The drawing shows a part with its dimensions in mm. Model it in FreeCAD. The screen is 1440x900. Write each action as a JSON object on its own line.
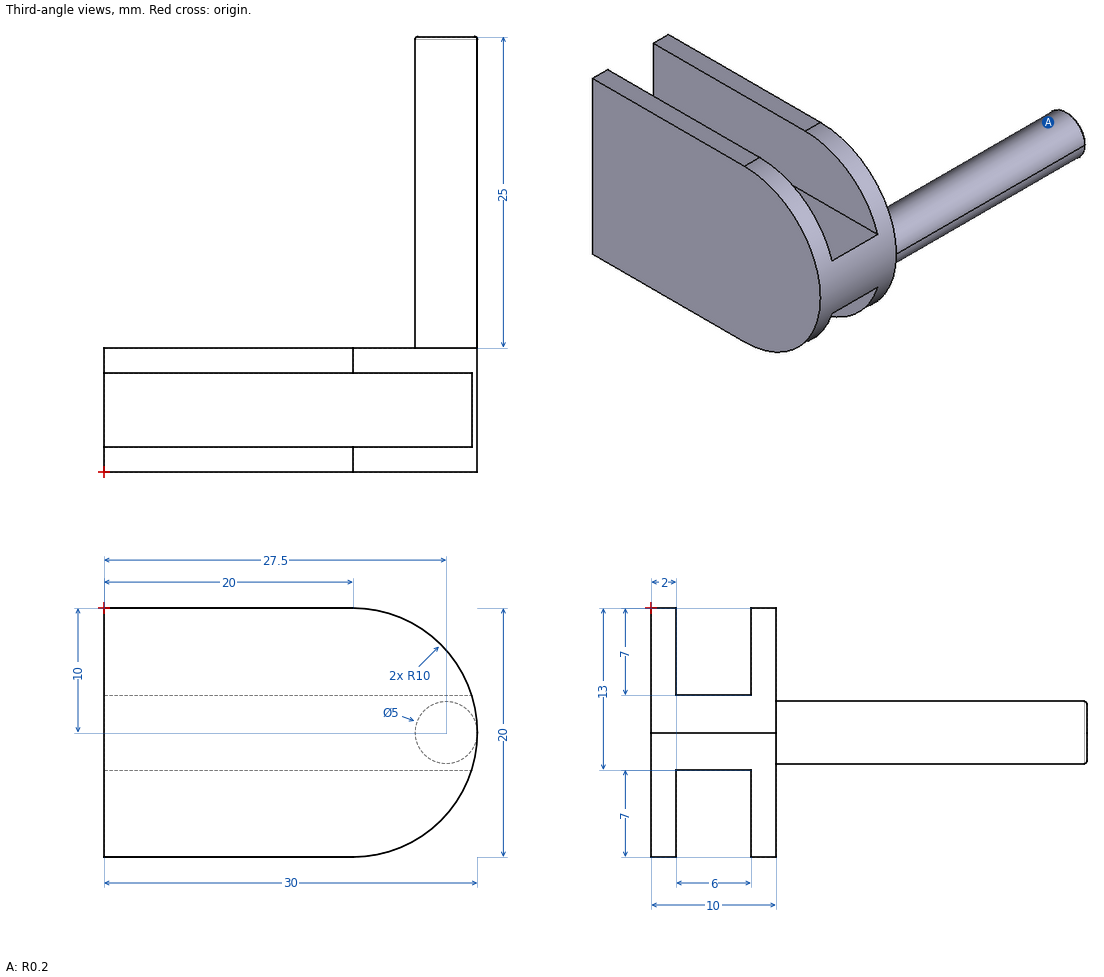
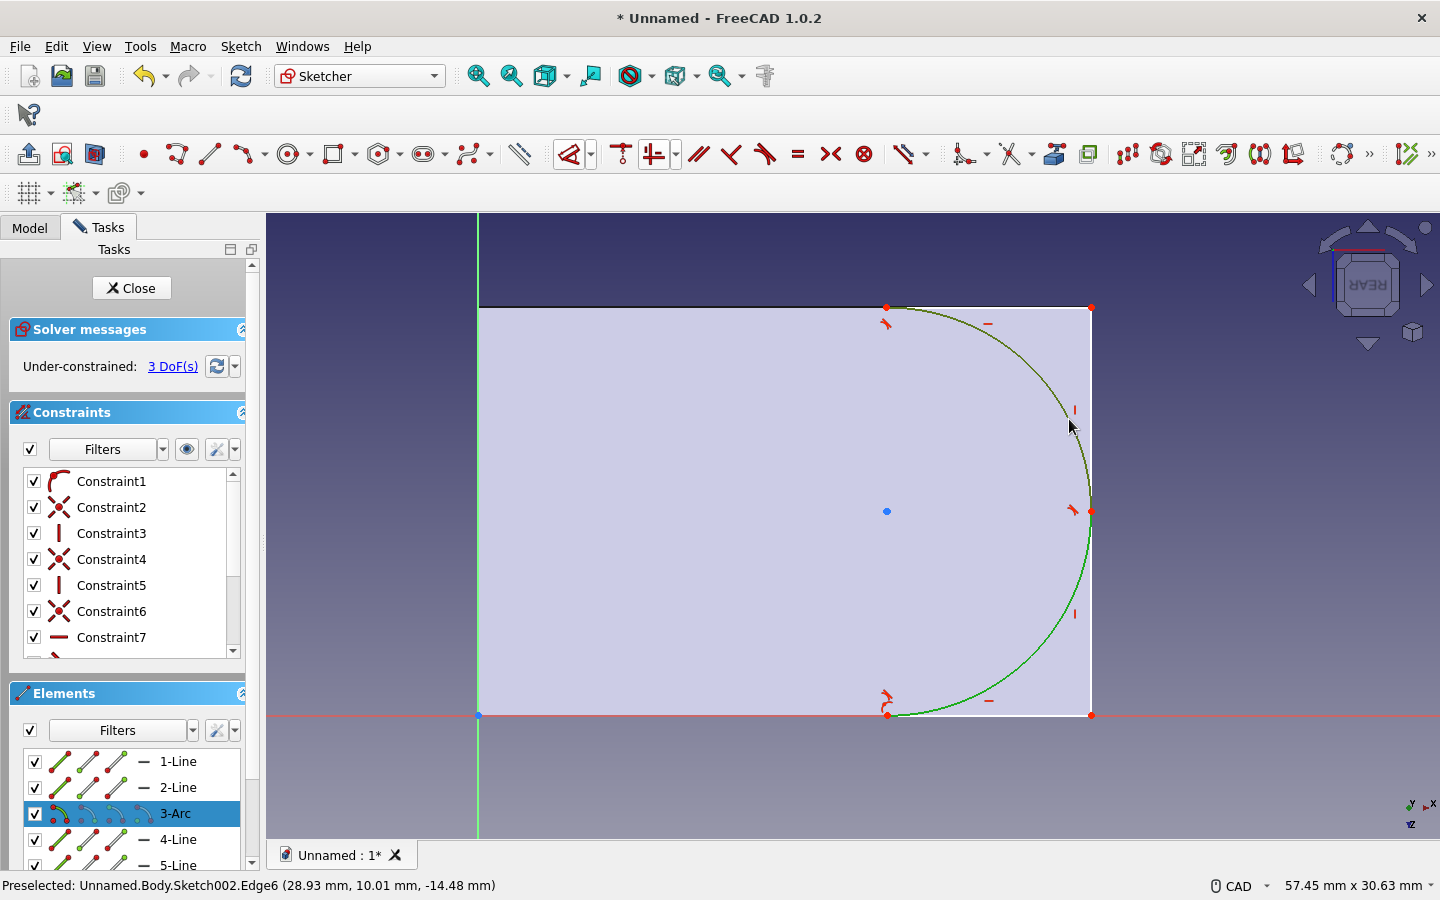
{"action": "left_click", "coordinate": [798, 154]}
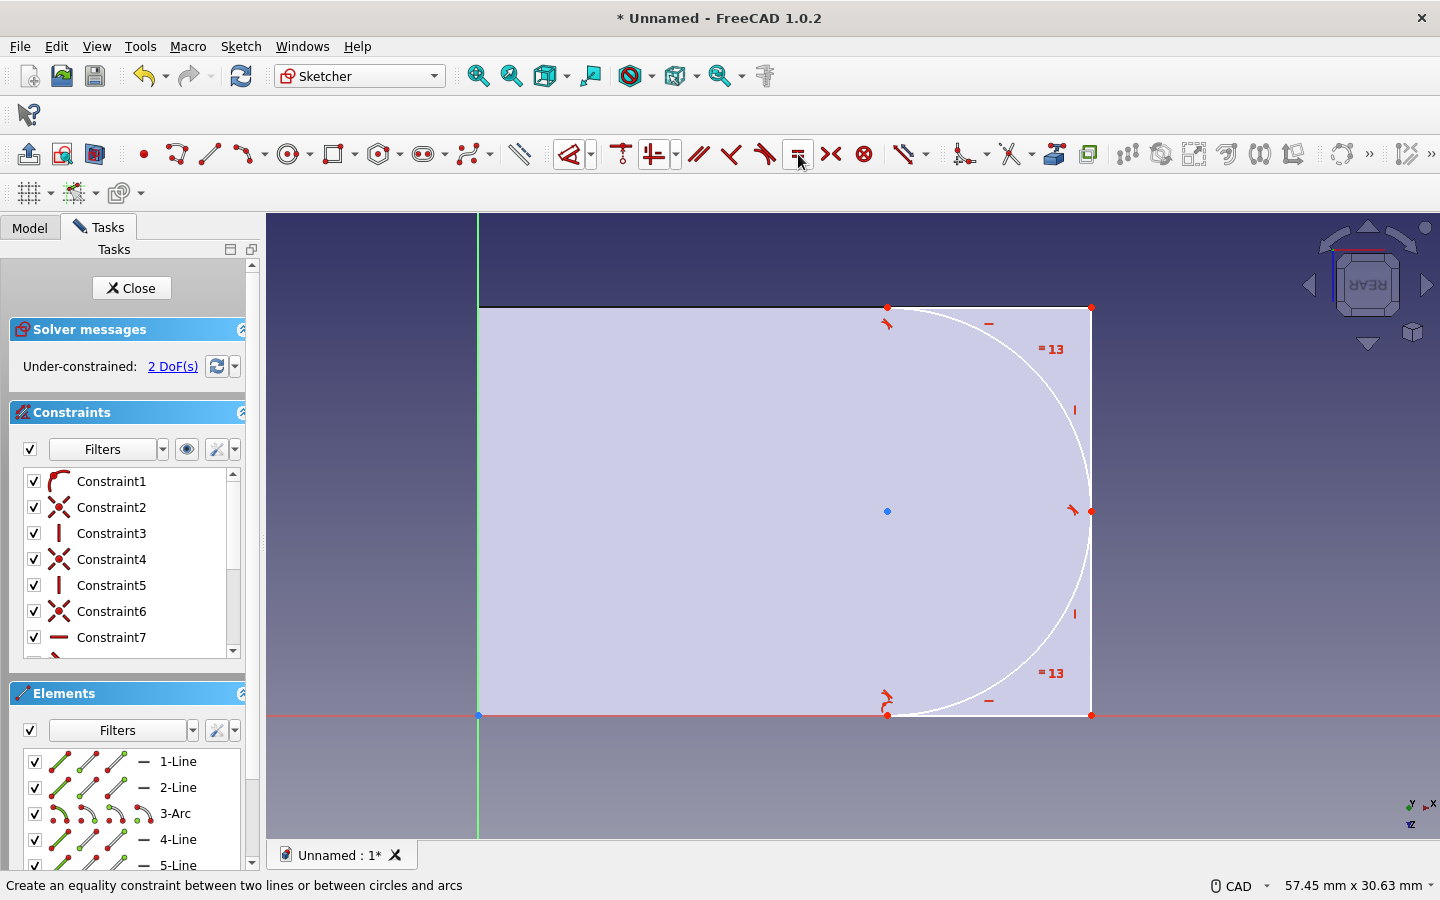
{"action": "left_click", "coordinate": [980, 694]}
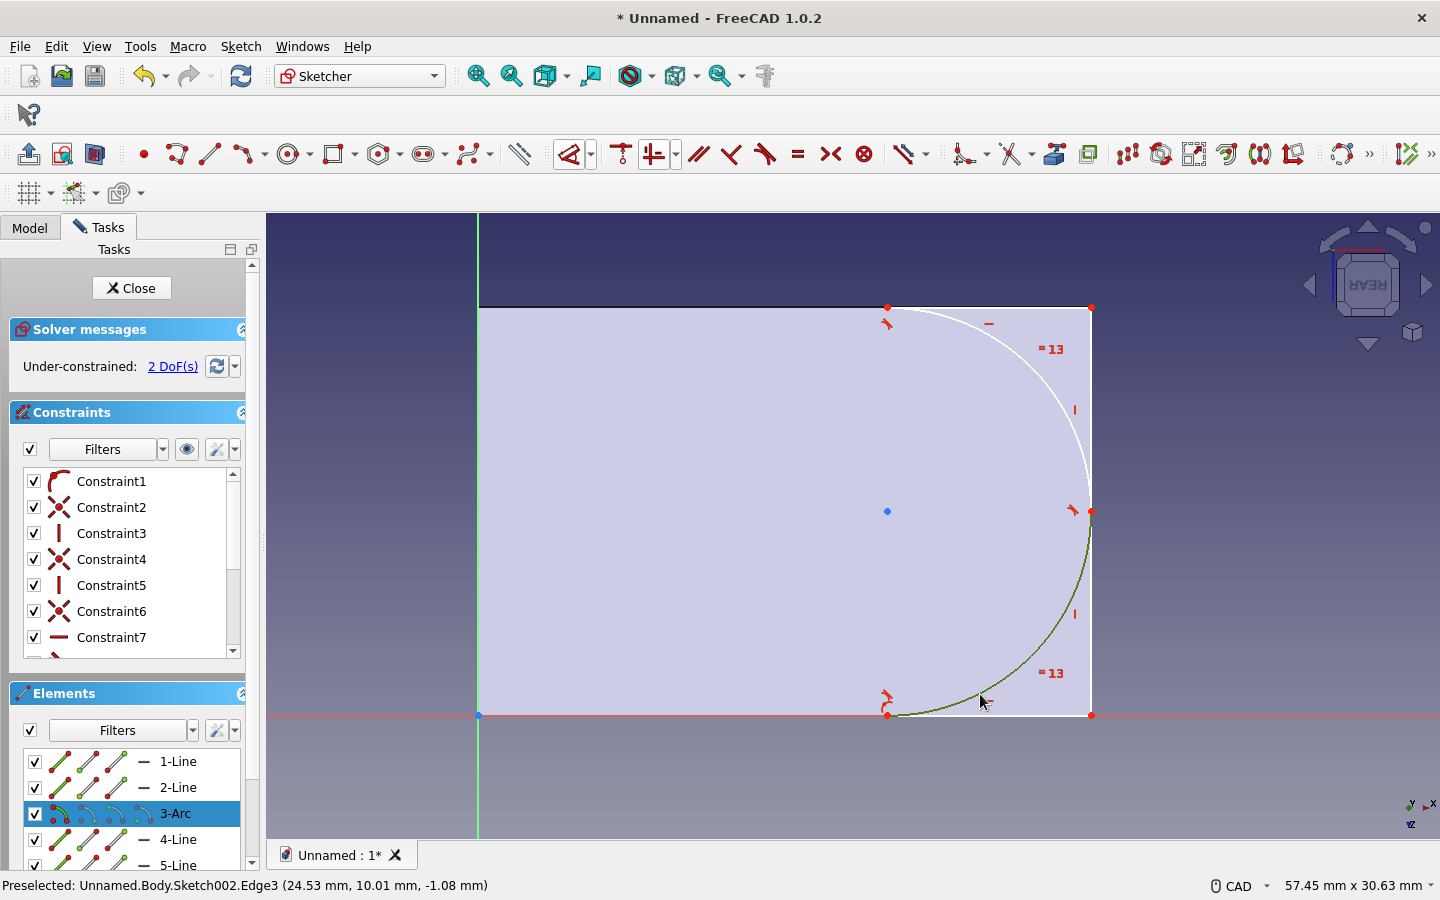
{"action": "key", "text": "k r"}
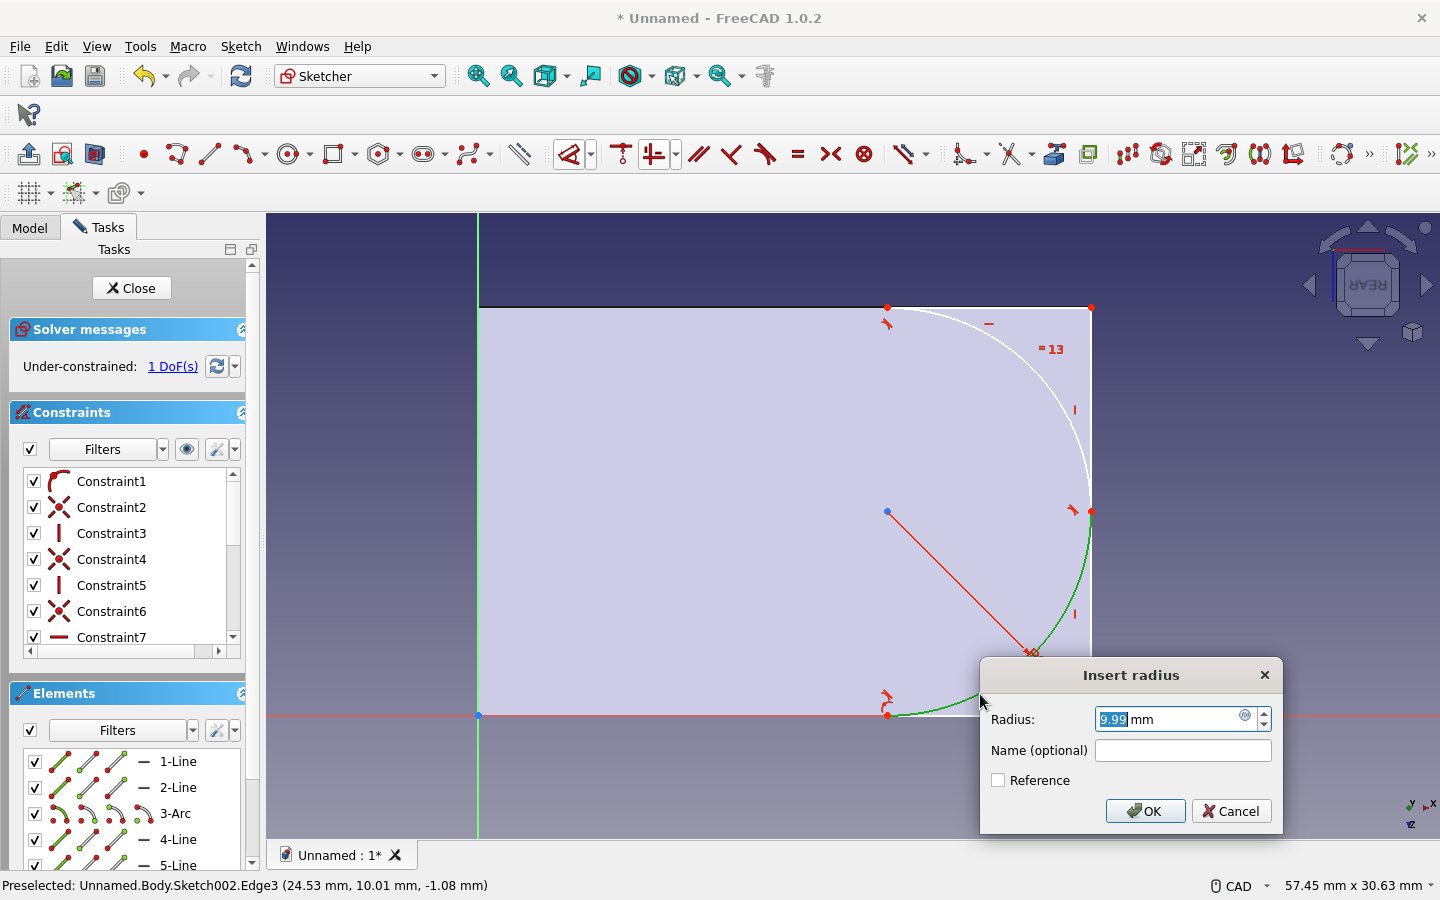
{"action": "type", "text": "10"}
{"action": "key", "text": "Return"}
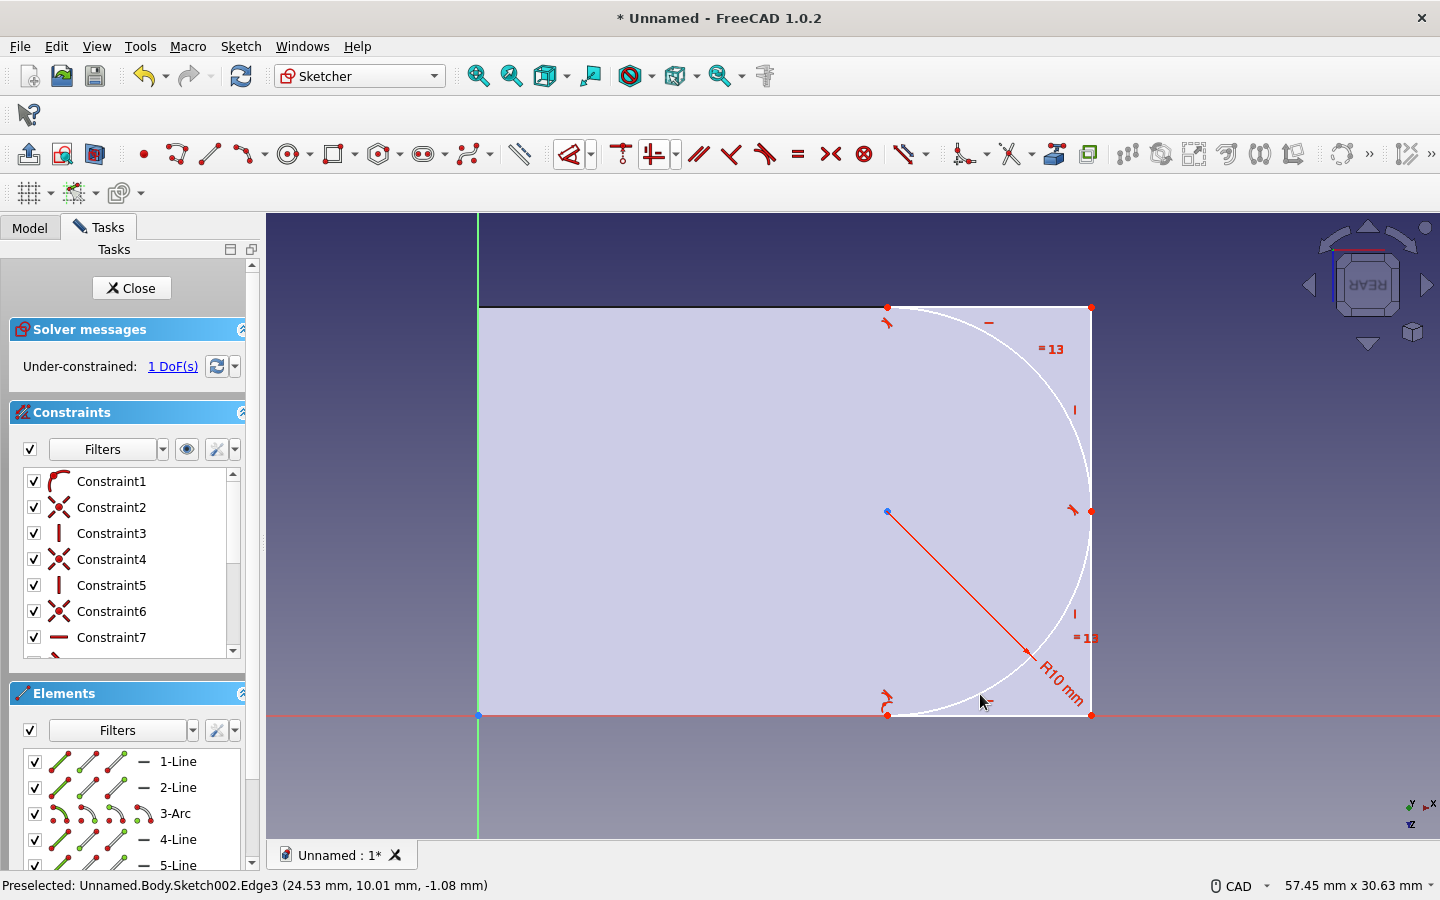
{"action": "left_click", "coordinate": [887, 716]}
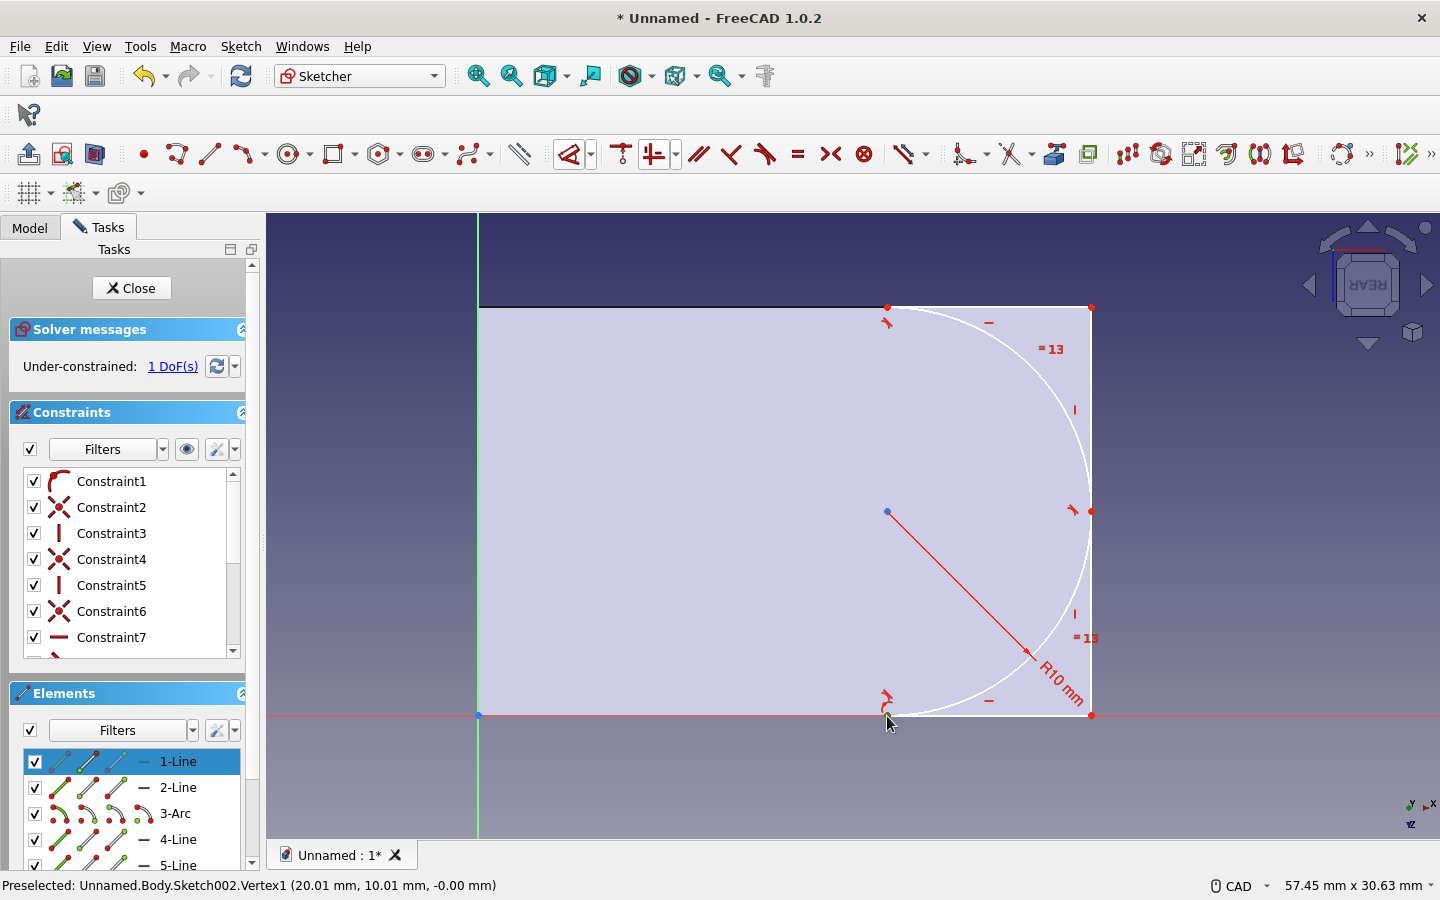
{"action": "key", "text": "l"}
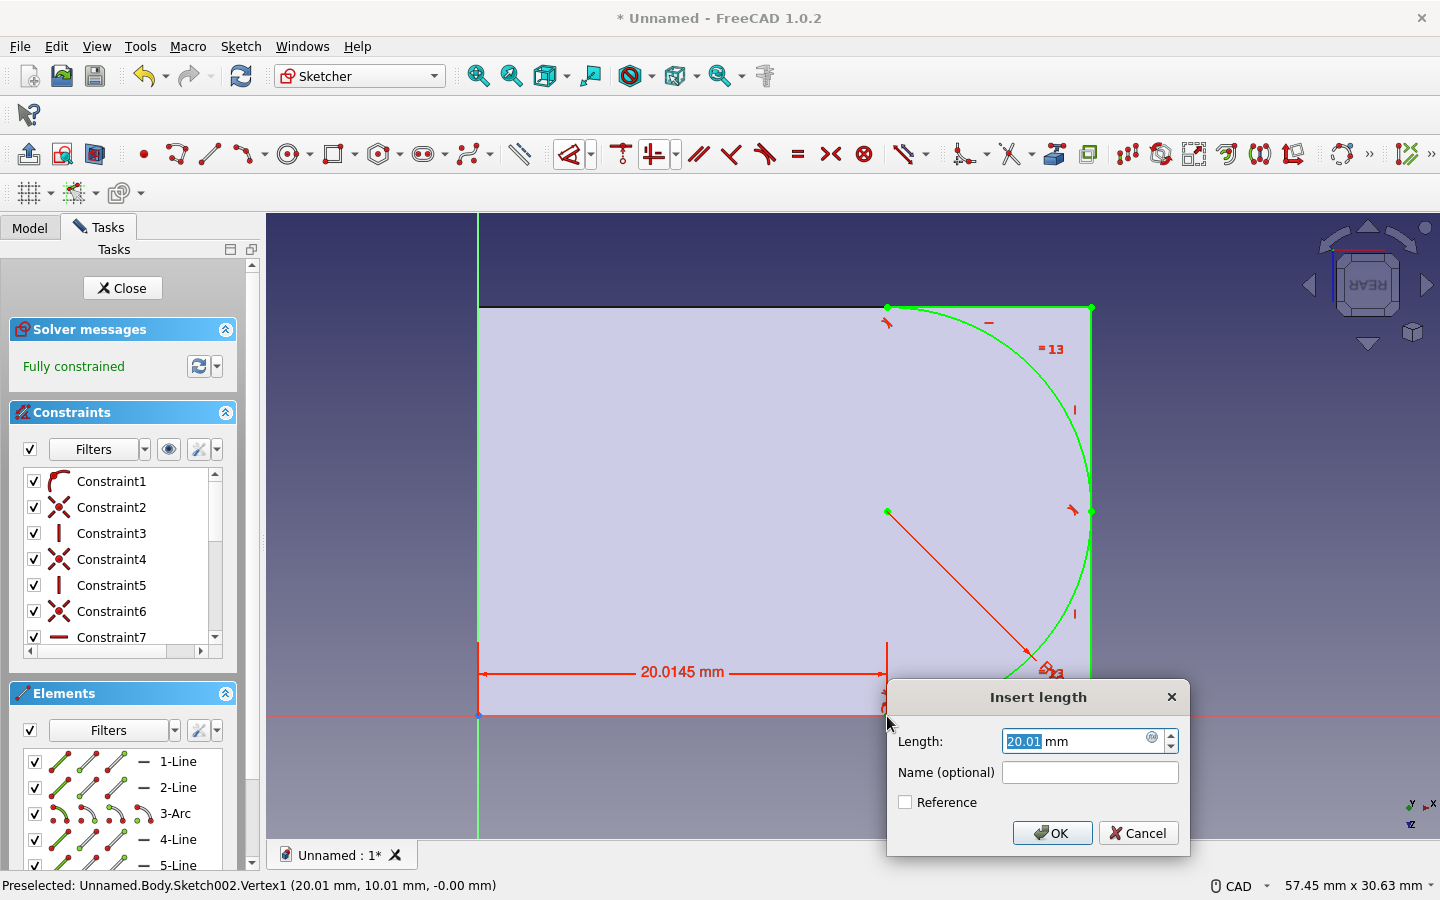
{"action": "type", "text": "20"}
{"action": "key", "text": "Return"}